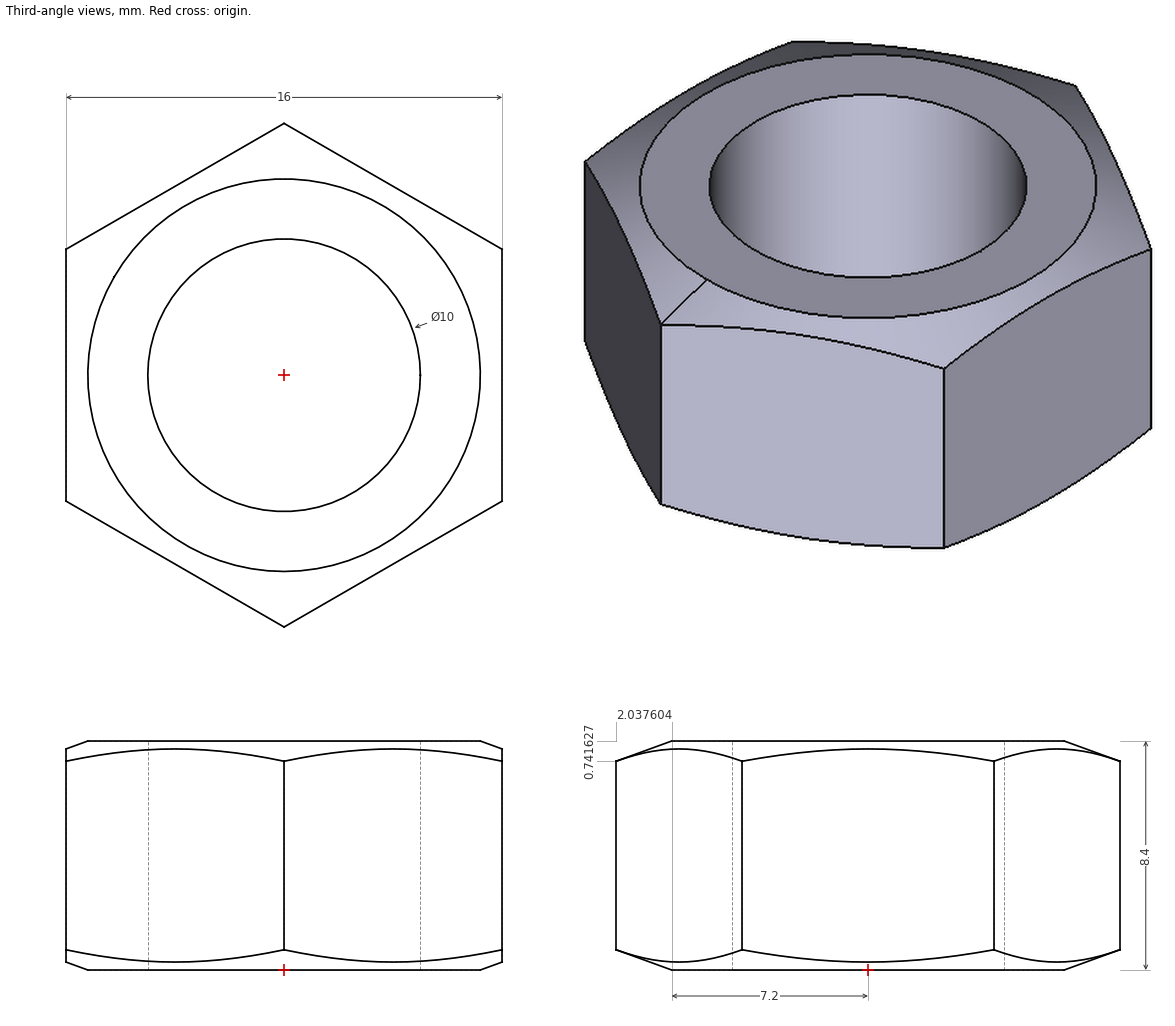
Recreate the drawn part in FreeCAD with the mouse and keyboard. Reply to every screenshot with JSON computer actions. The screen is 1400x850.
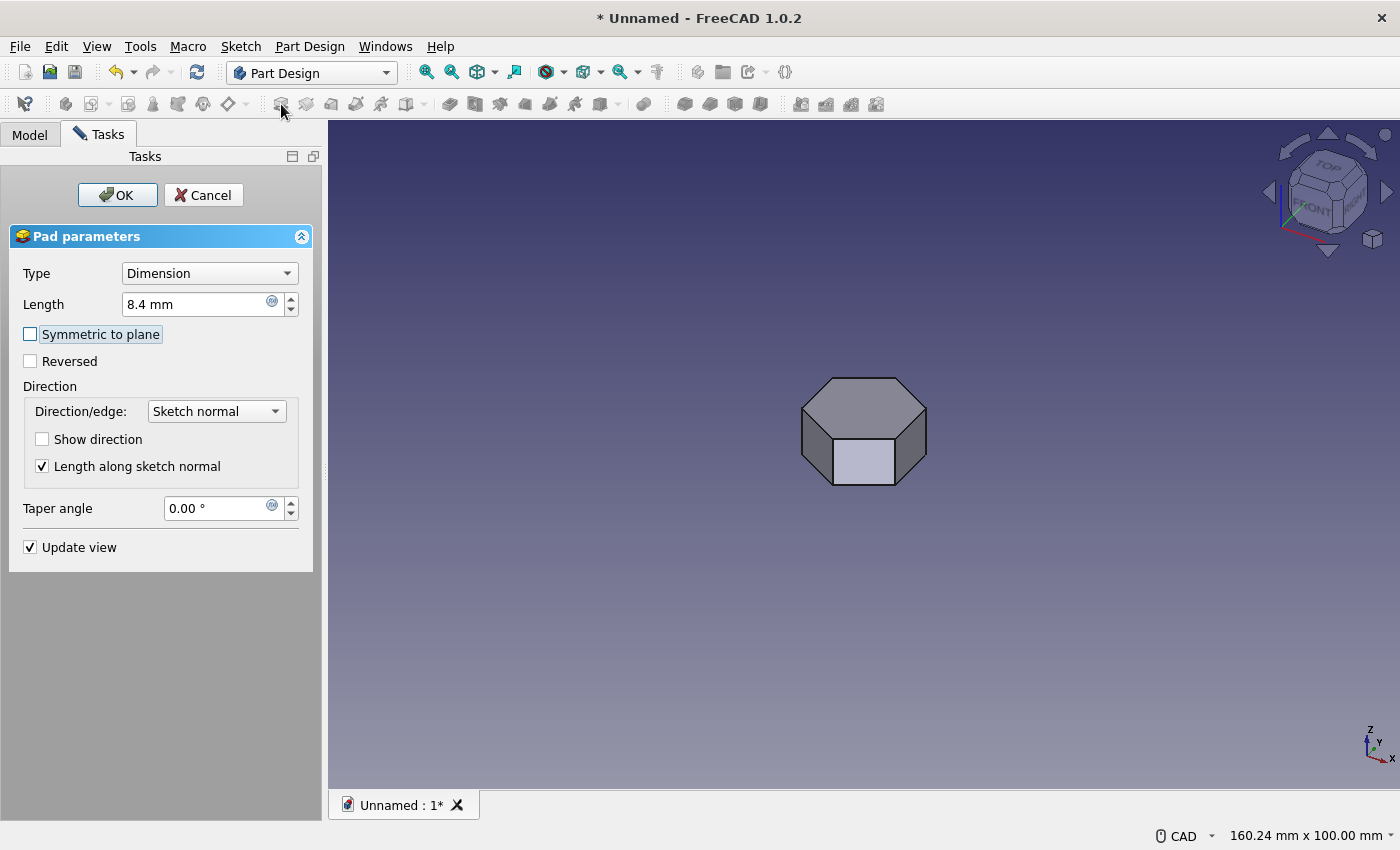
{"action": "left_click", "coordinate": [118, 195]}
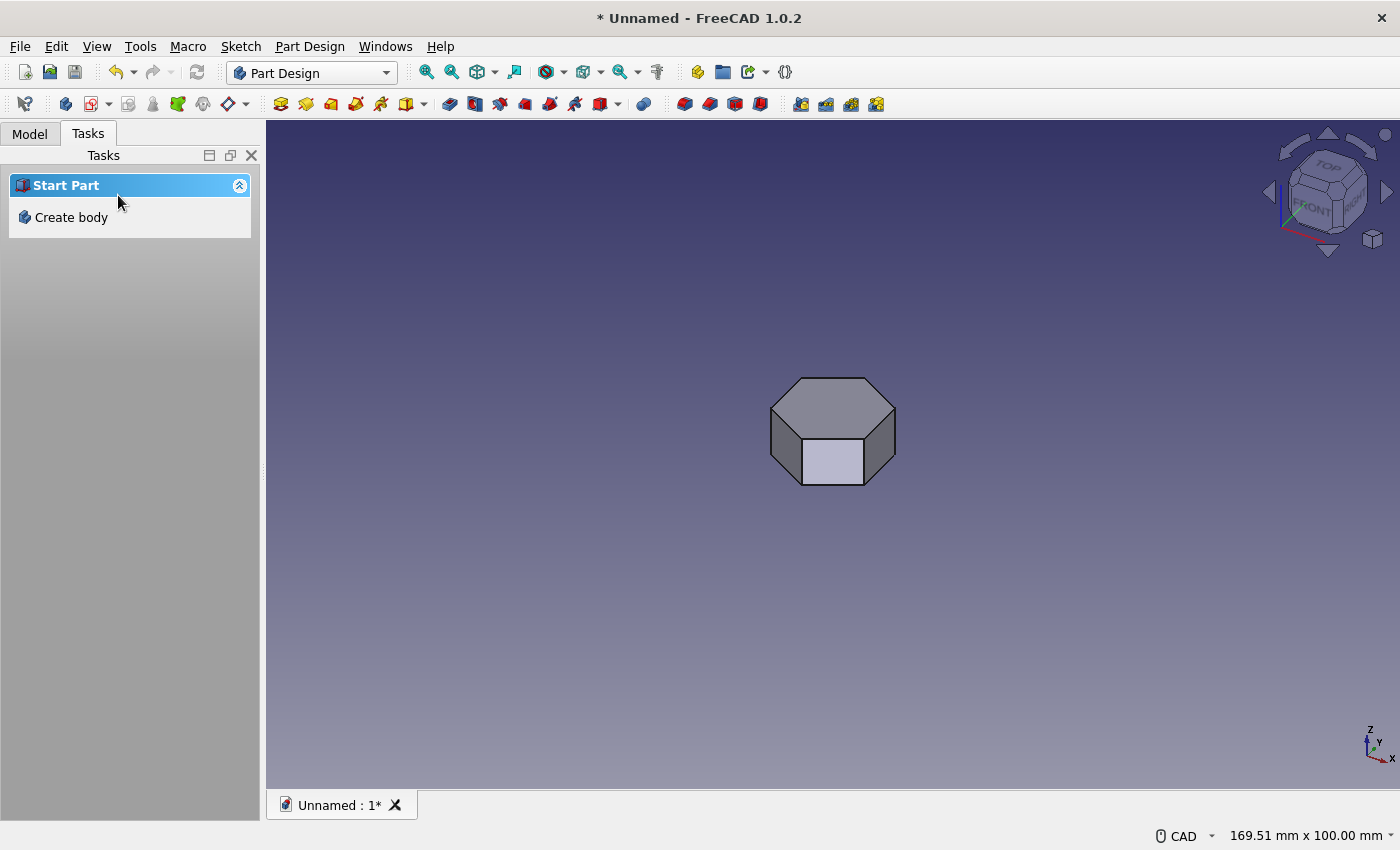
{"action": "left_click", "coordinate": [427, 72]}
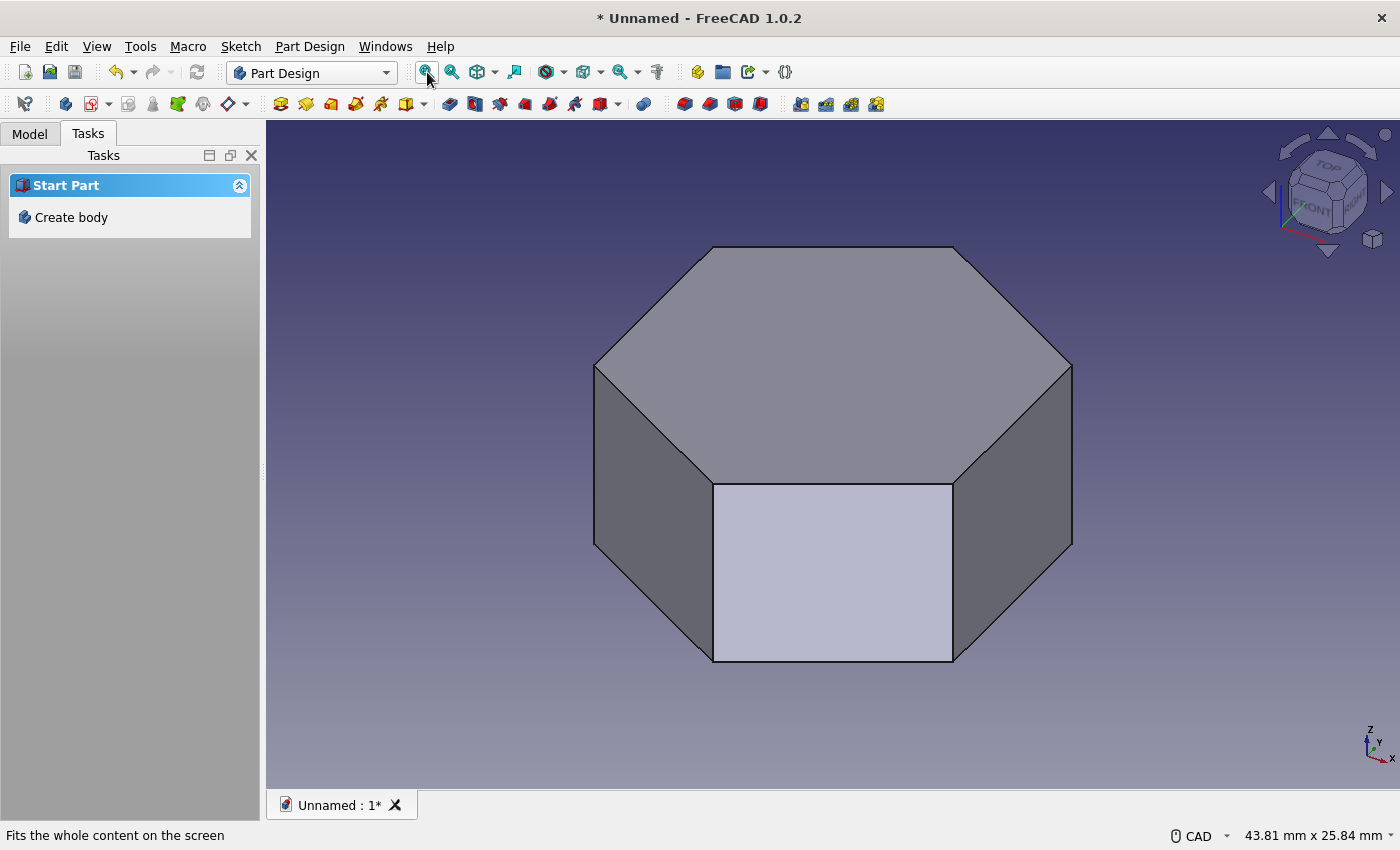
{"action": "left_click", "coordinate": [90, 104]}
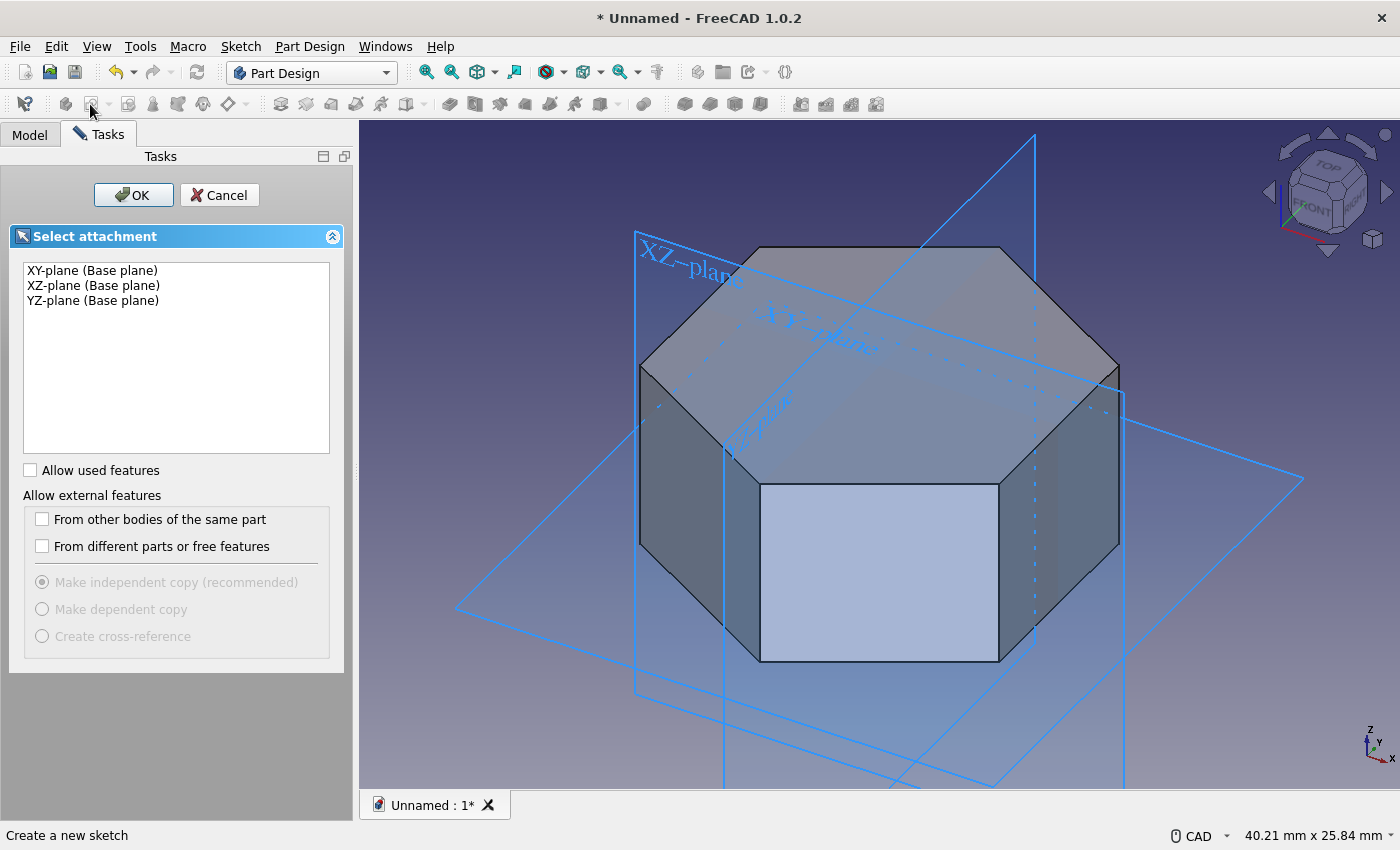
{"action": "left_click", "coordinate": [84, 300]}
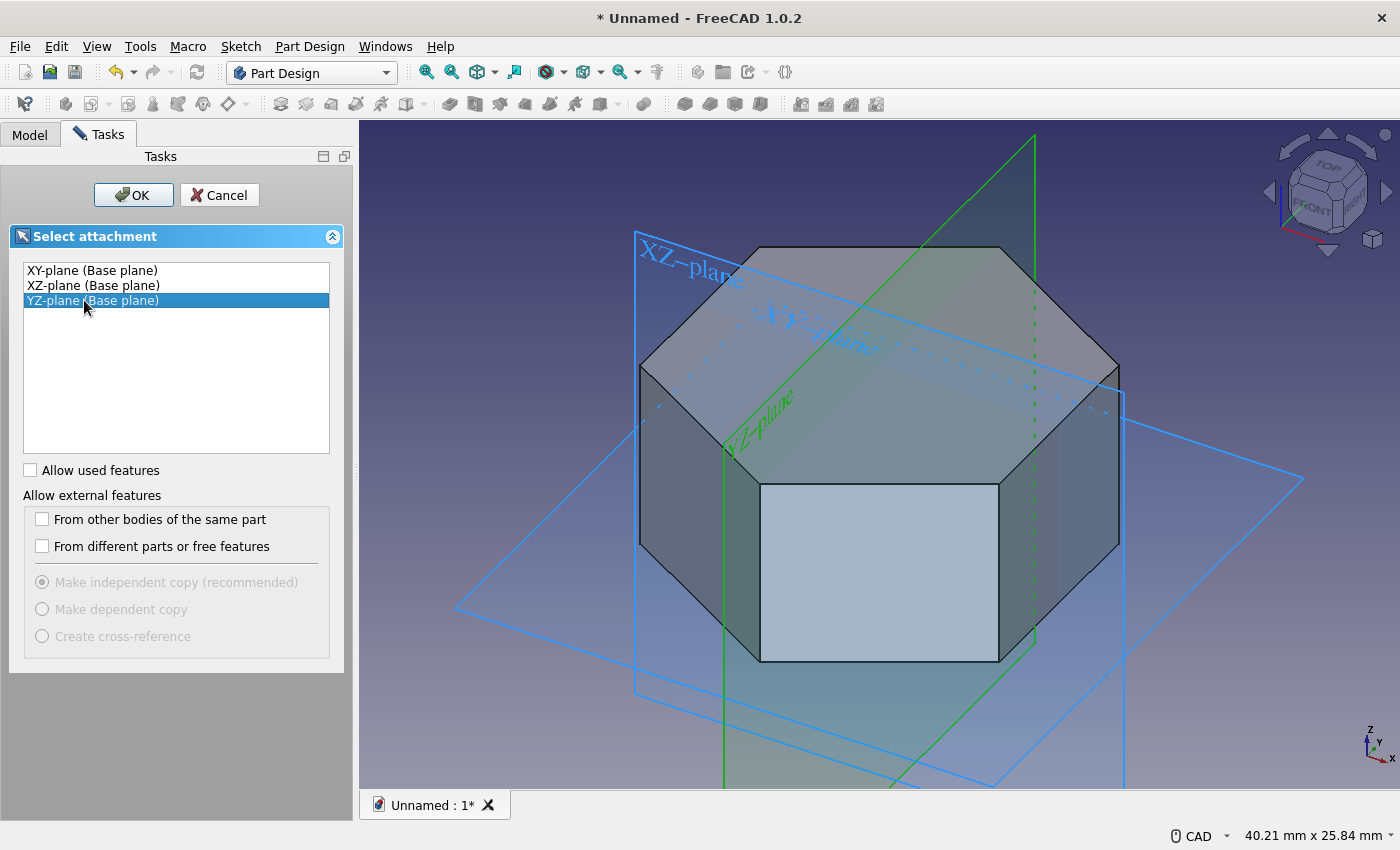
{"action": "left_click", "coordinate": [134, 195]}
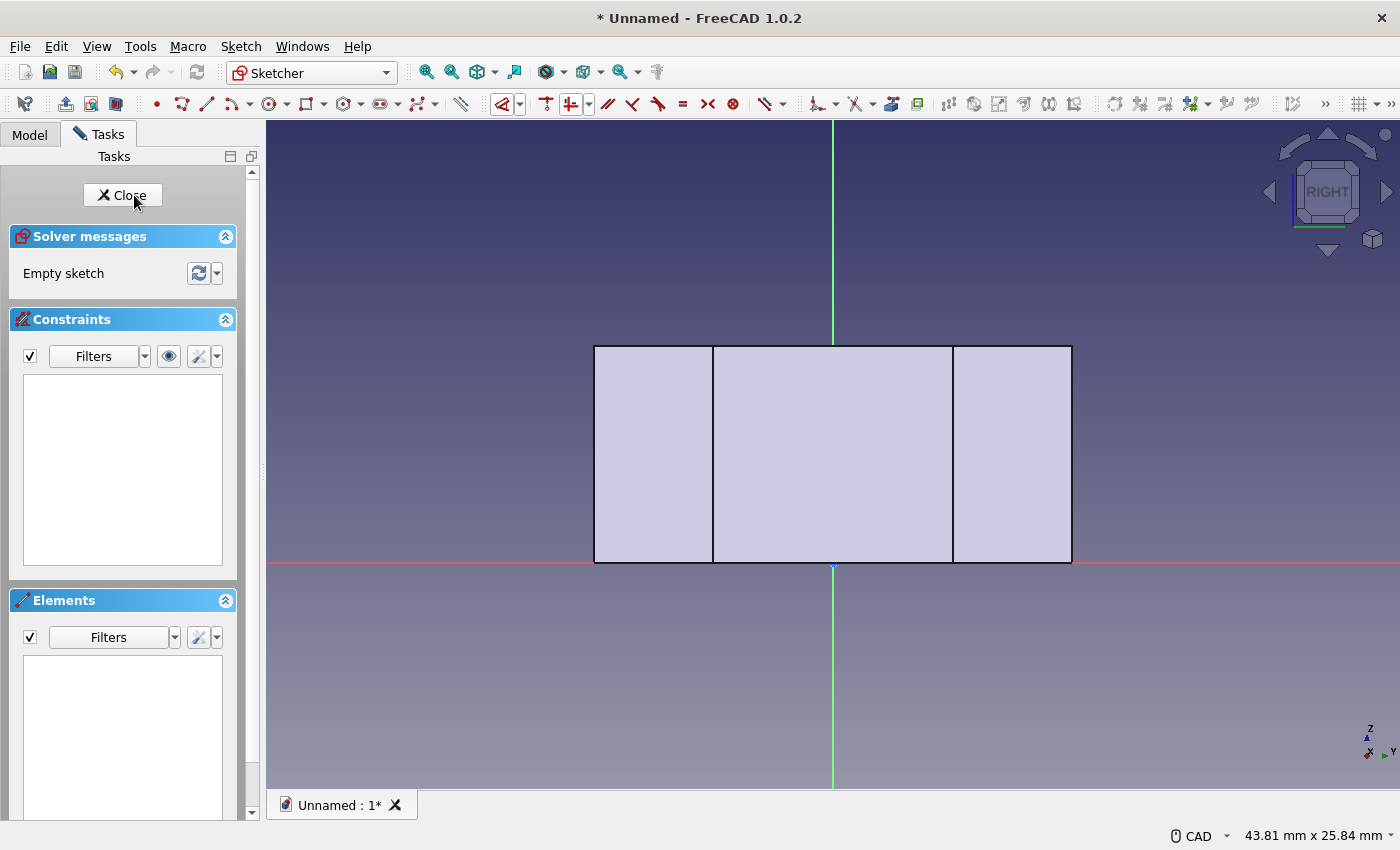
{"action": "left_click", "coordinate": [116, 104]}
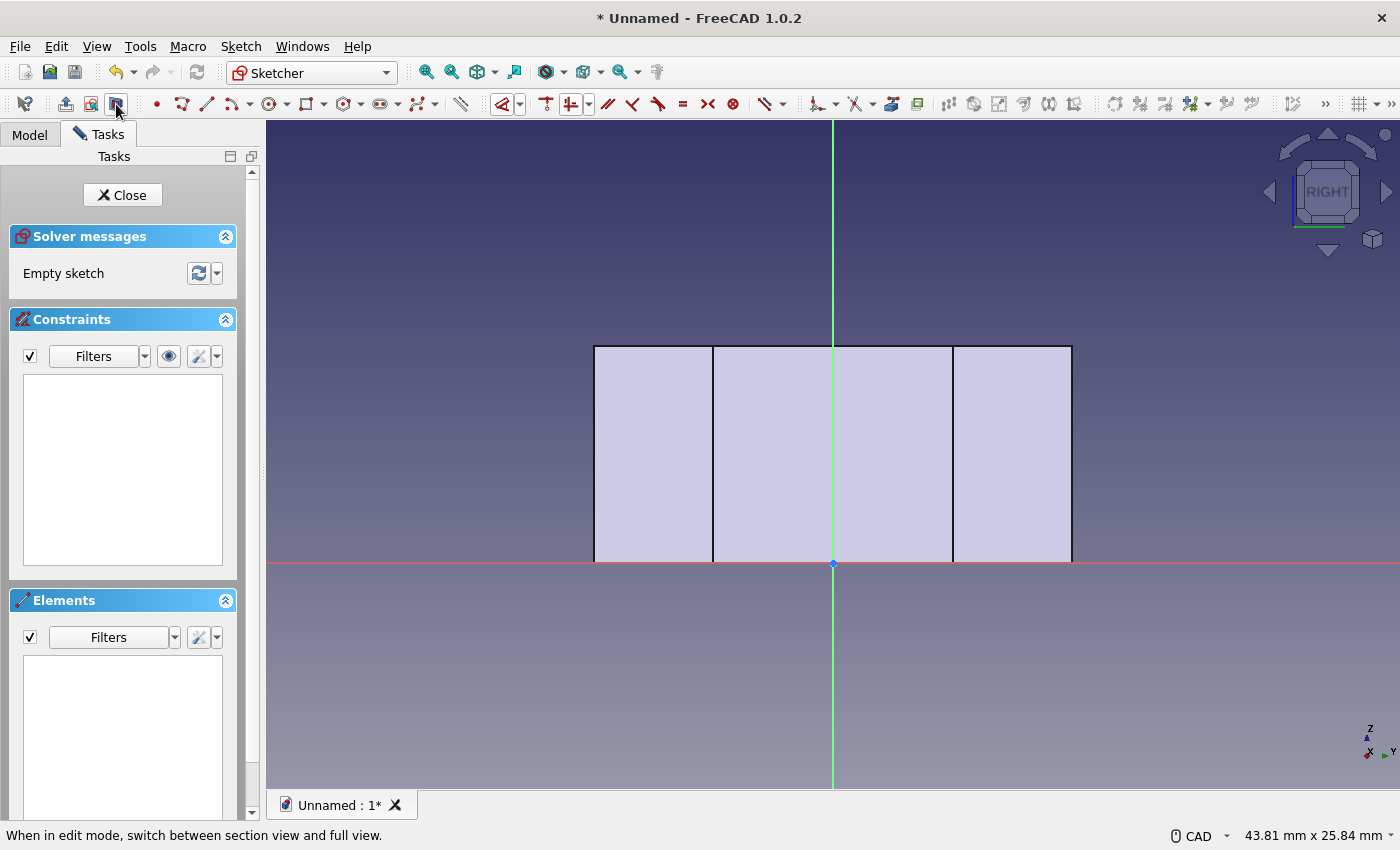
{"action": "scroll", "coordinate": [609, 347], "scroll_direction": "up", "scroll_amount": 13}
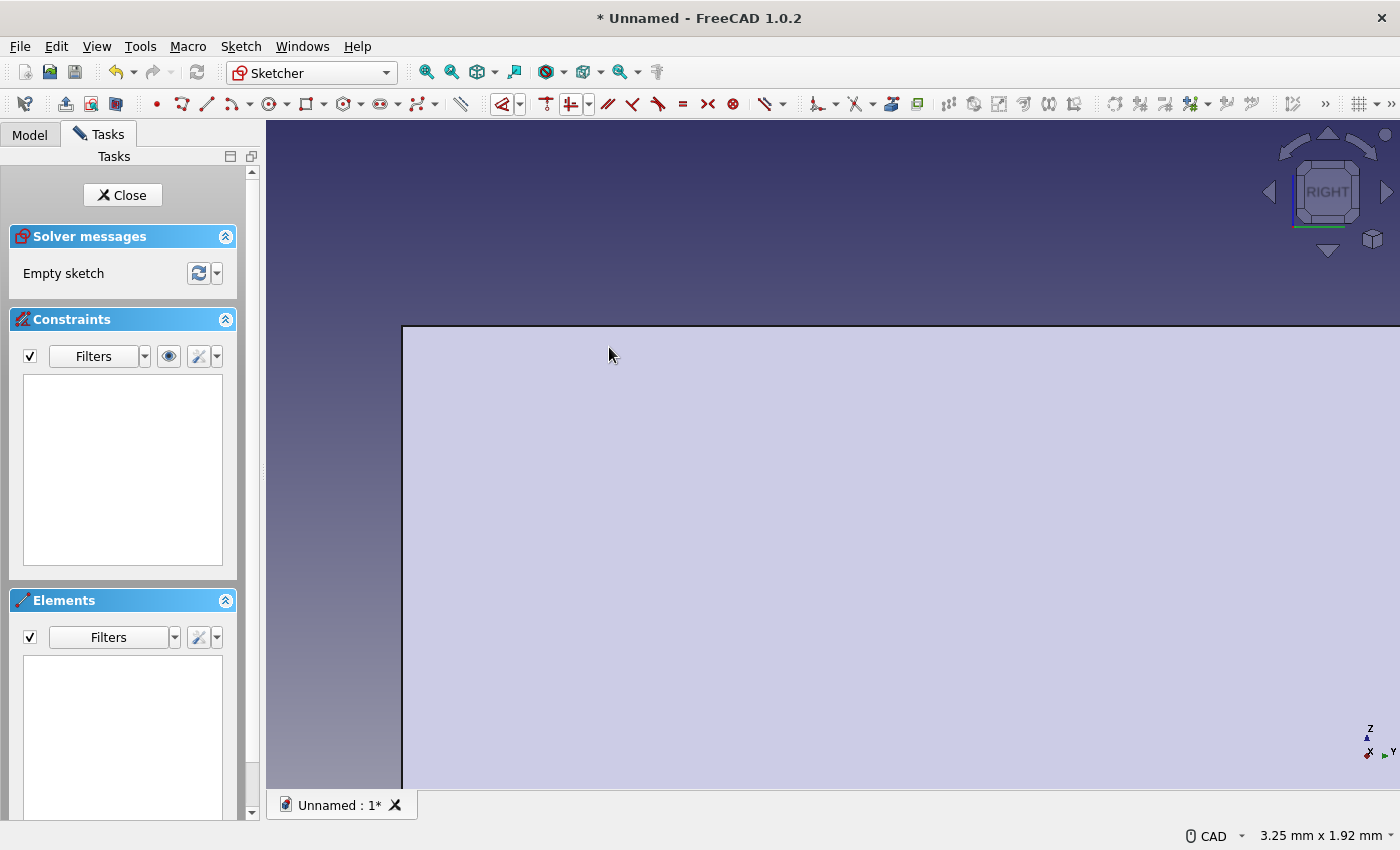
{"action": "left_click", "coordinate": [182, 104]}